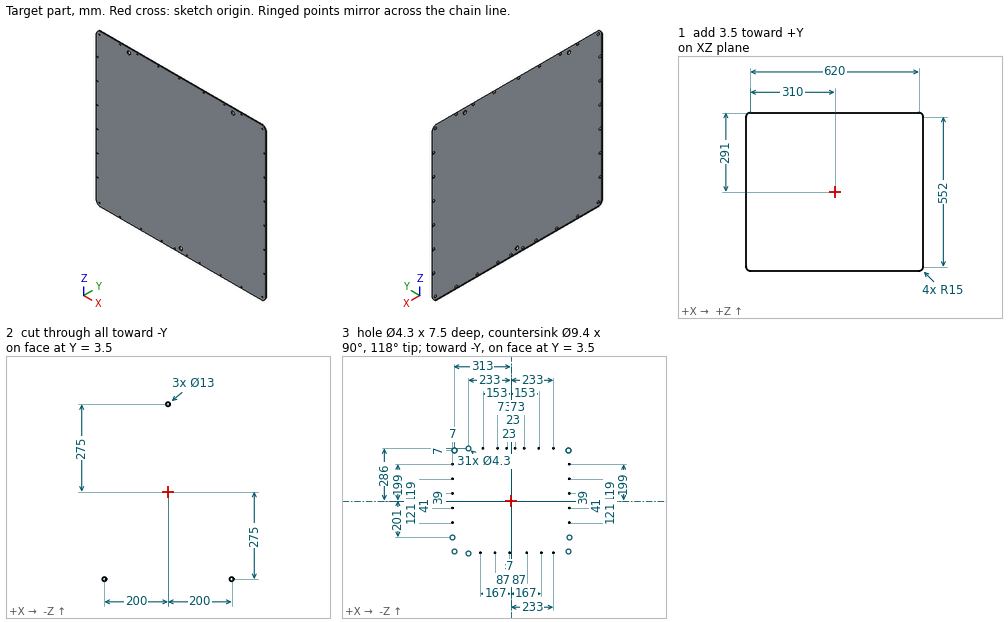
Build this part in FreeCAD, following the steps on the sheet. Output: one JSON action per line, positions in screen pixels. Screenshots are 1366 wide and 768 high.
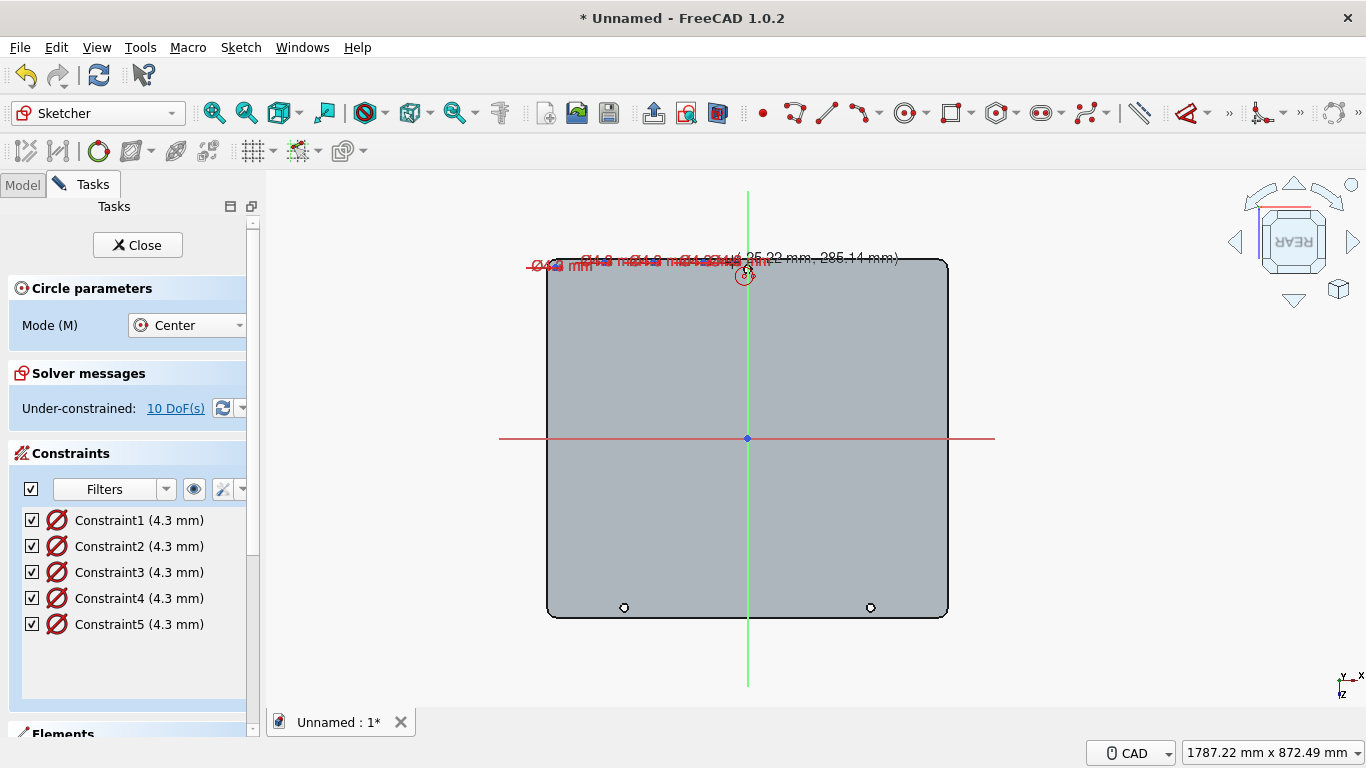
{"action": "scroll", "coordinate": [792, 262], "scroll_direction": "up", "scroll_amount": 15}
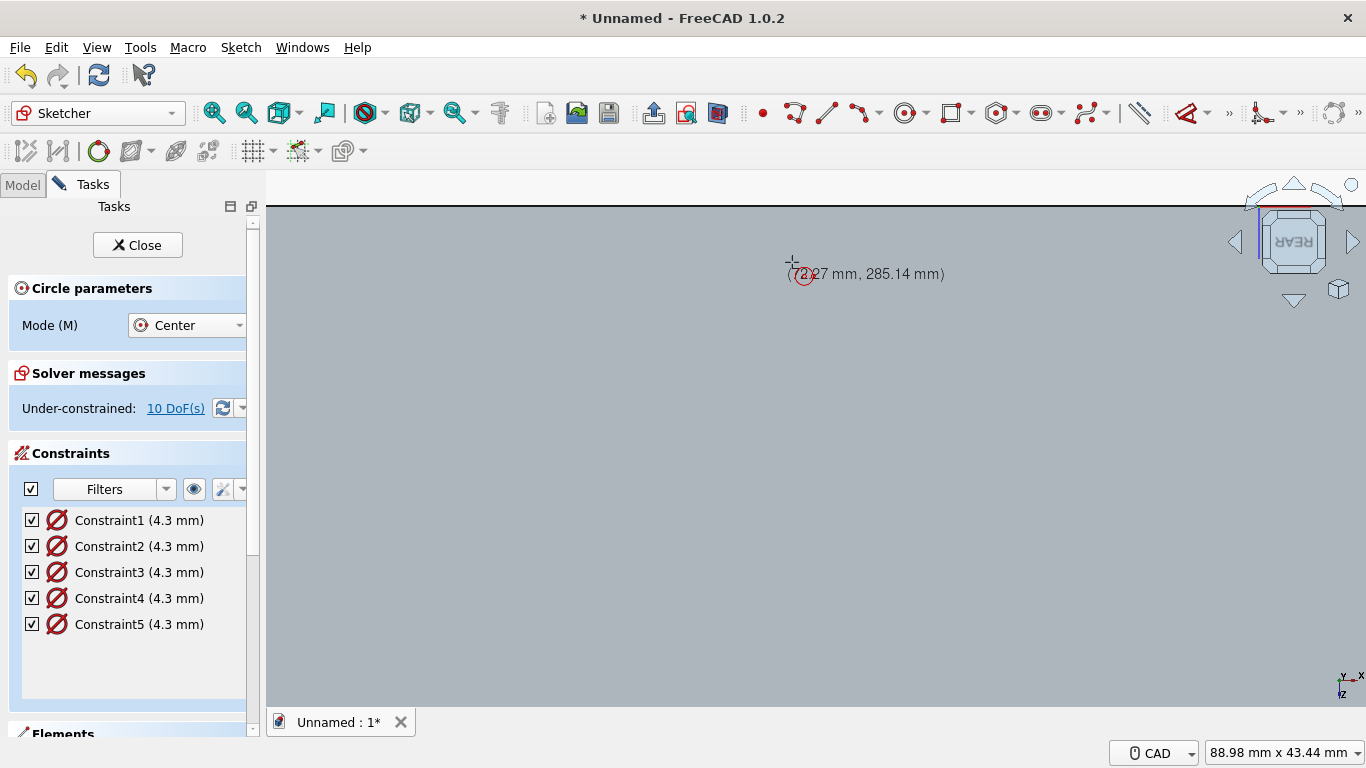
{"action": "scroll", "coordinate": [792, 262], "scroll_direction": "down", "scroll_amount": 15}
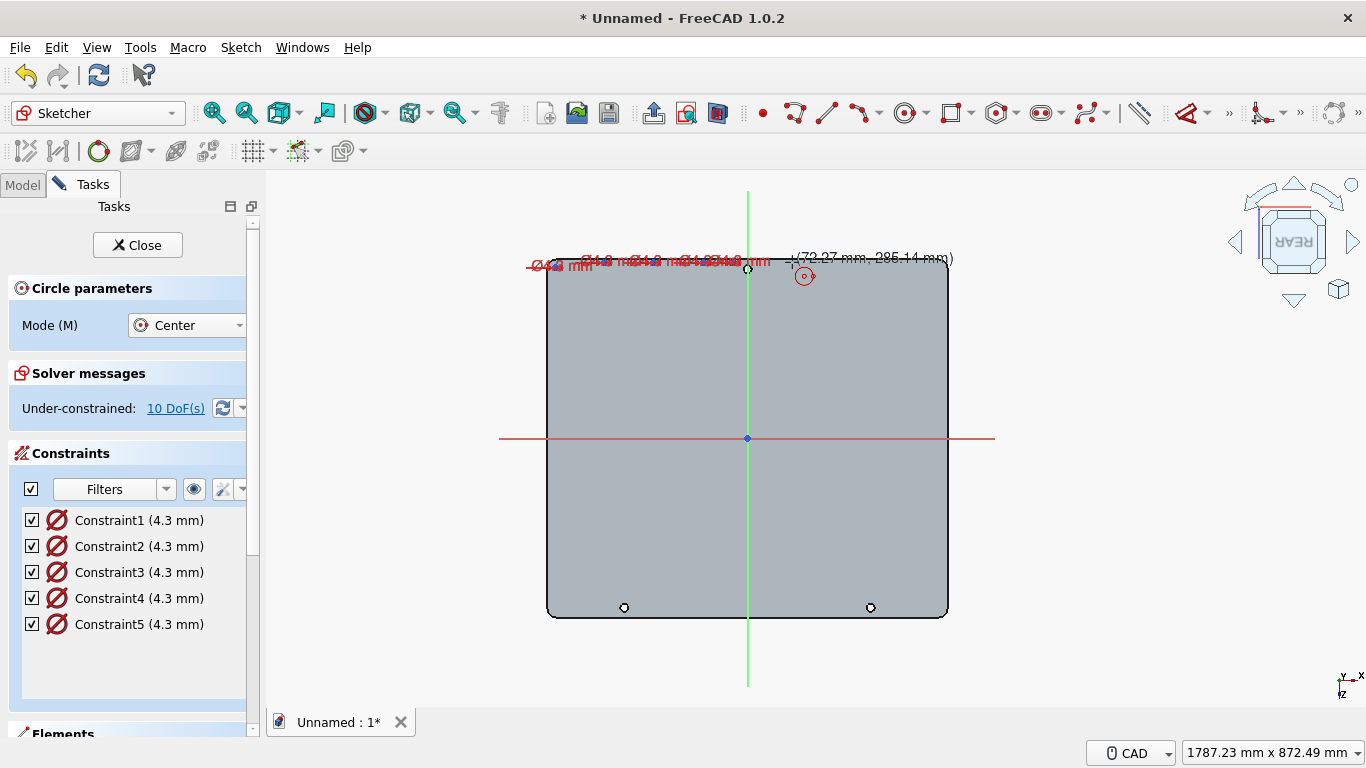
{"action": "left_click", "coordinate": [792, 262]}
{"action": "mouse_move", "coordinate": [793, 262]}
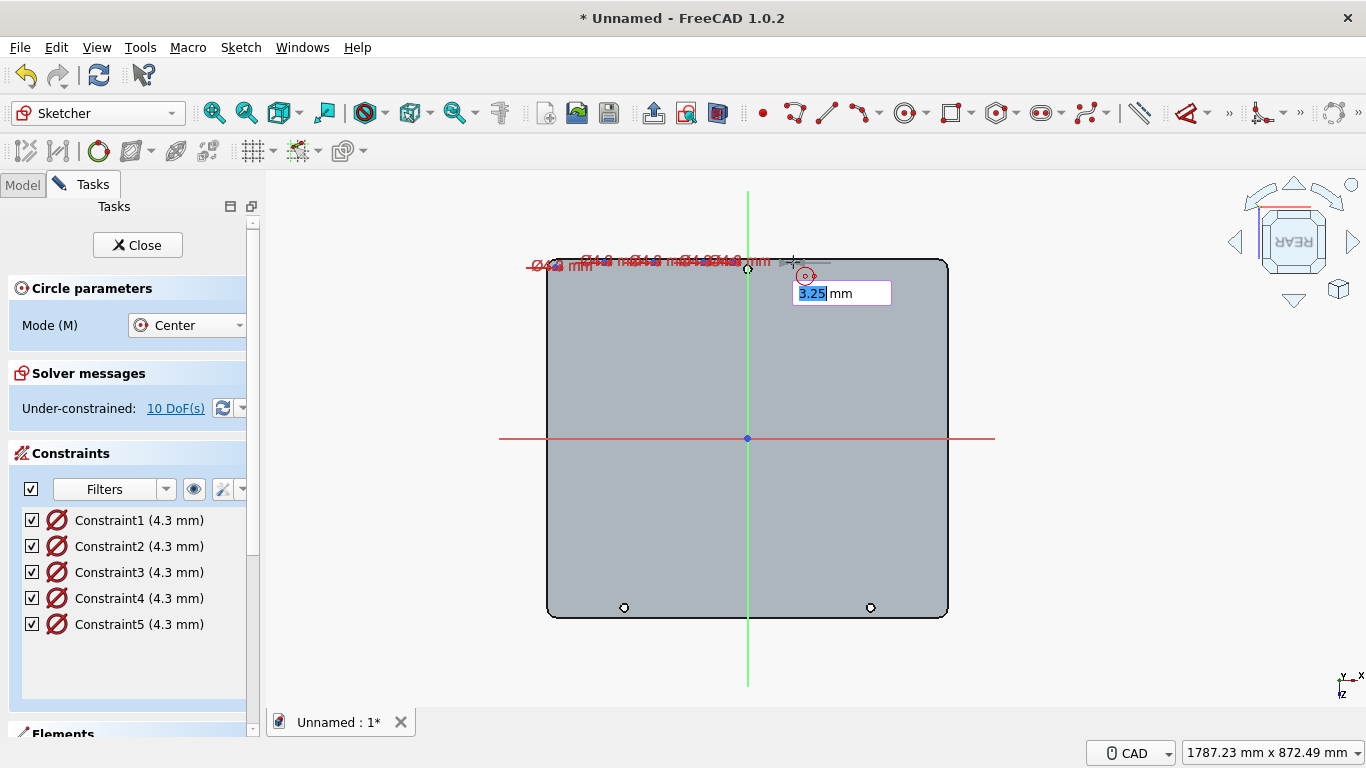
{"action": "type", "text": "4.3"}
{"action": "key", "text": "Return"}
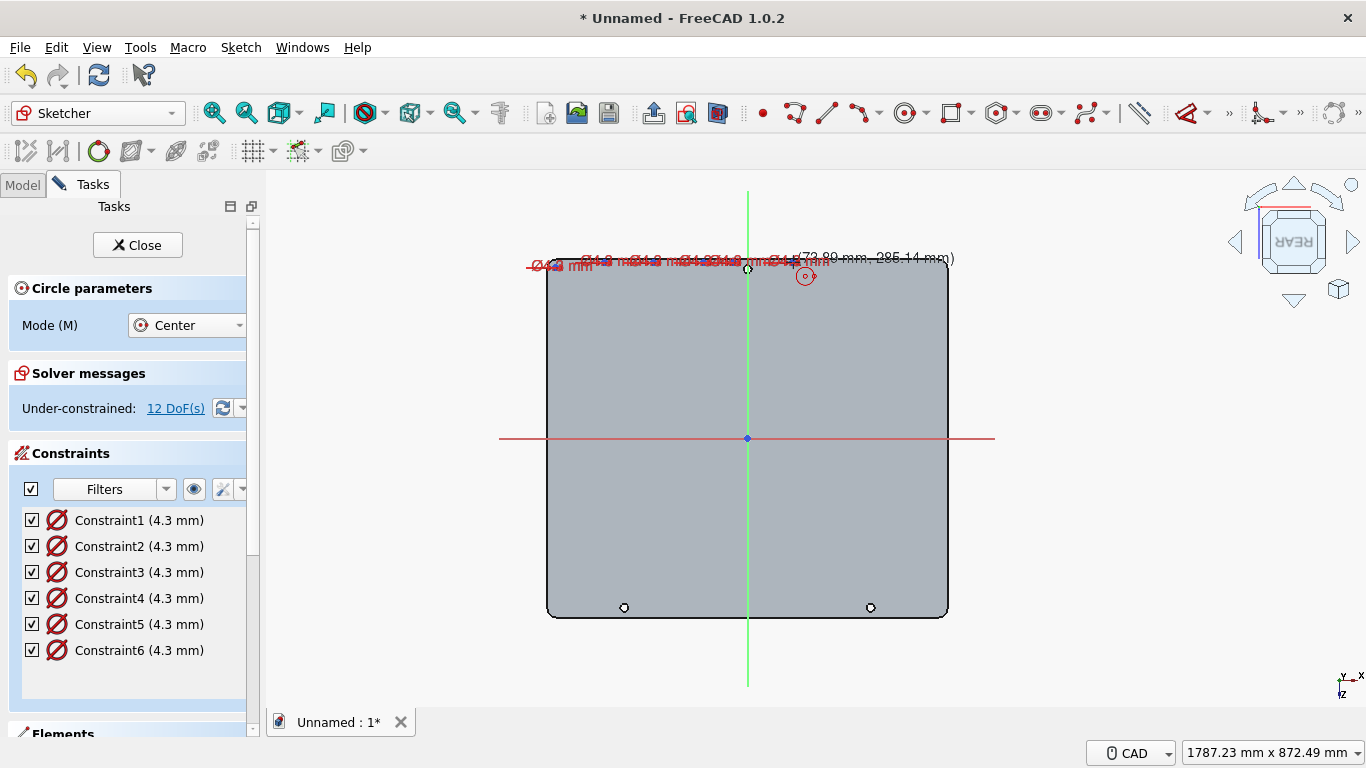
{"action": "scroll", "coordinate": [842, 262], "scroll_direction": "up", "scroll_amount": 15}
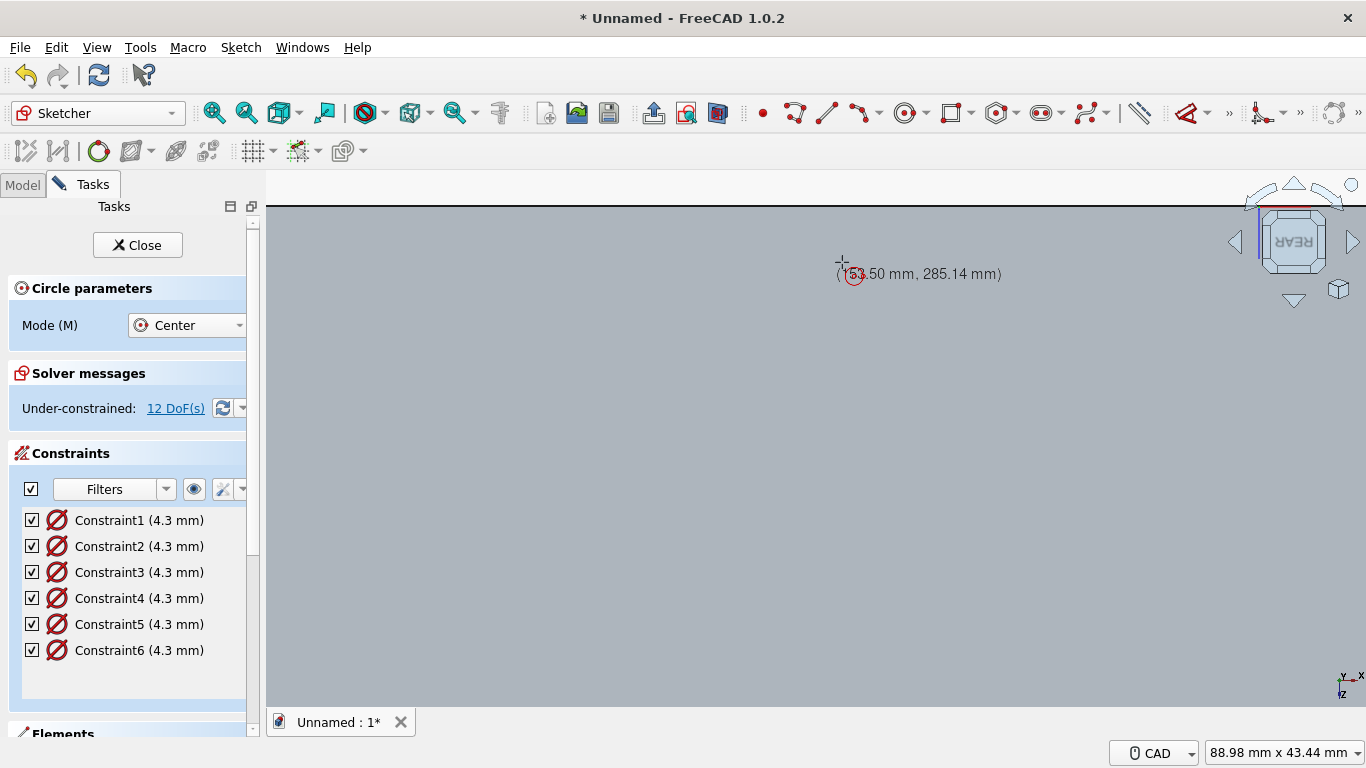
{"action": "scroll", "coordinate": [843, 262], "scroll_direction": "down", "scroll_amount": 15}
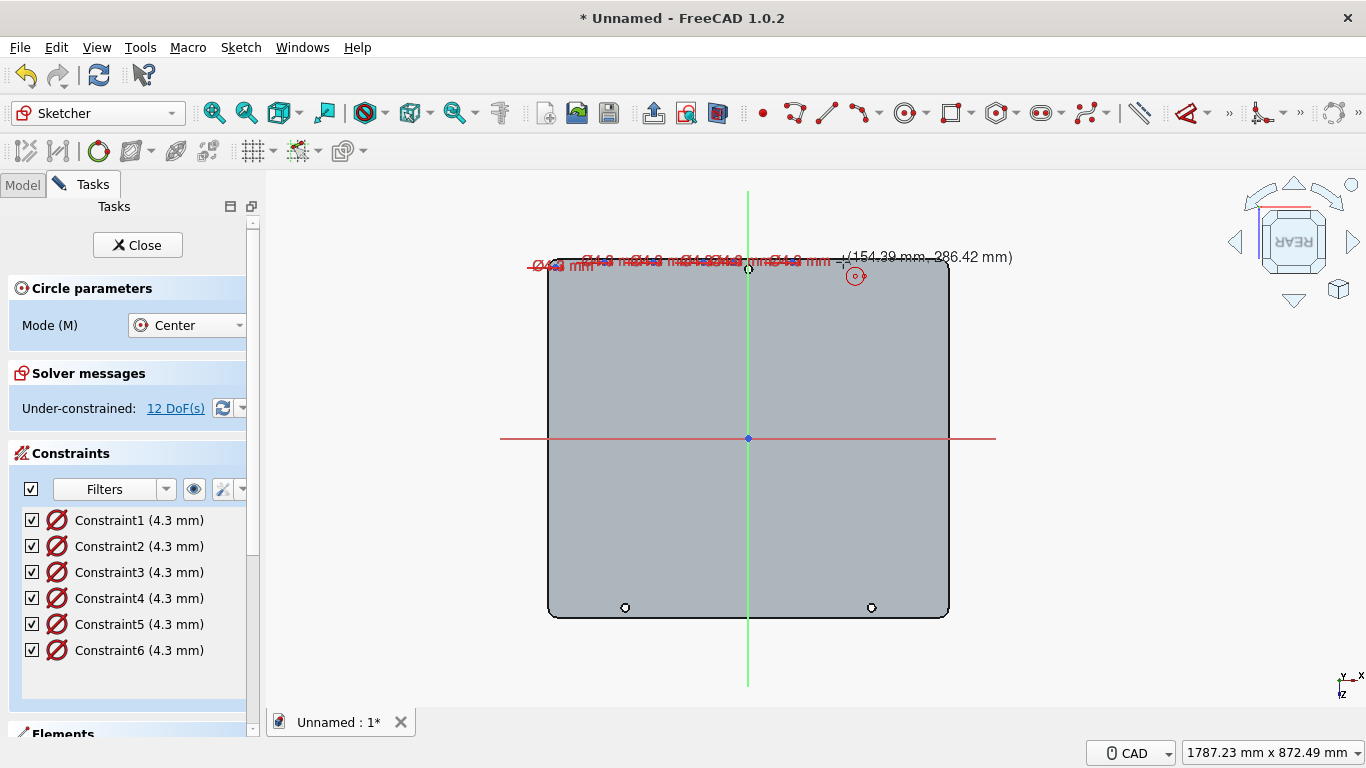
{"action": "left_click", "coordinate": [843, 262]}
{"action": "mouse_move", "coordinate": [844, 262]}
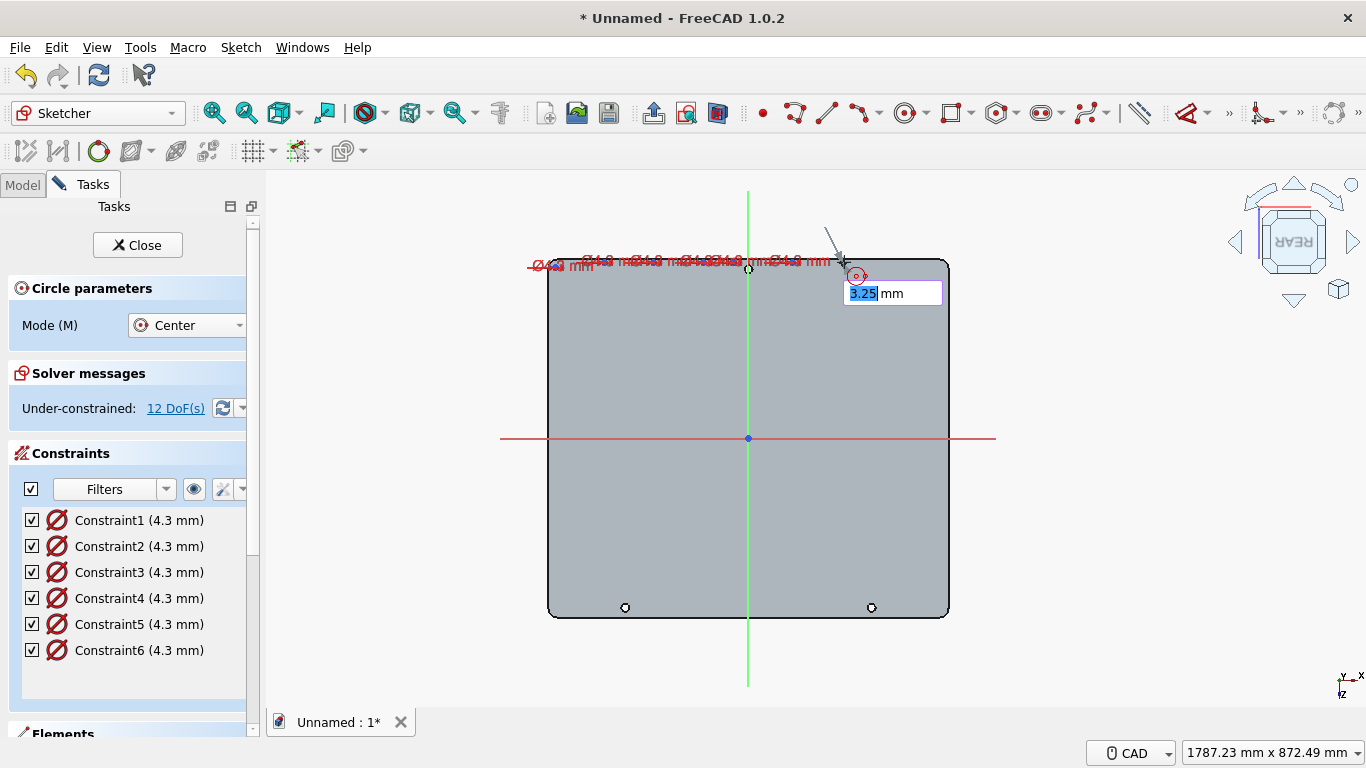
{"action": "type", "text": "4.3"}
{"action": "key", "text": "Return"}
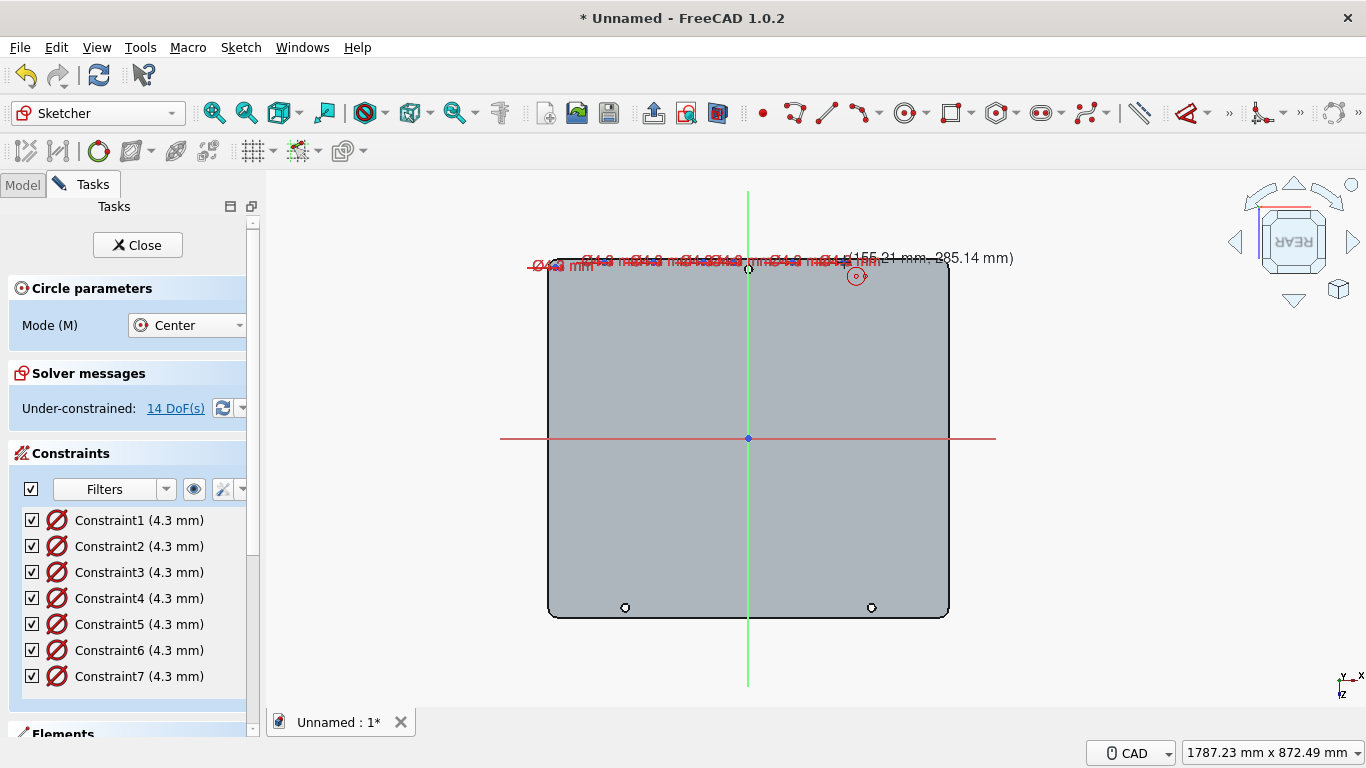
{"action": "scroll", "coordinate": [941, 267], "scroll_direction": "up", "scroll_amount": 15}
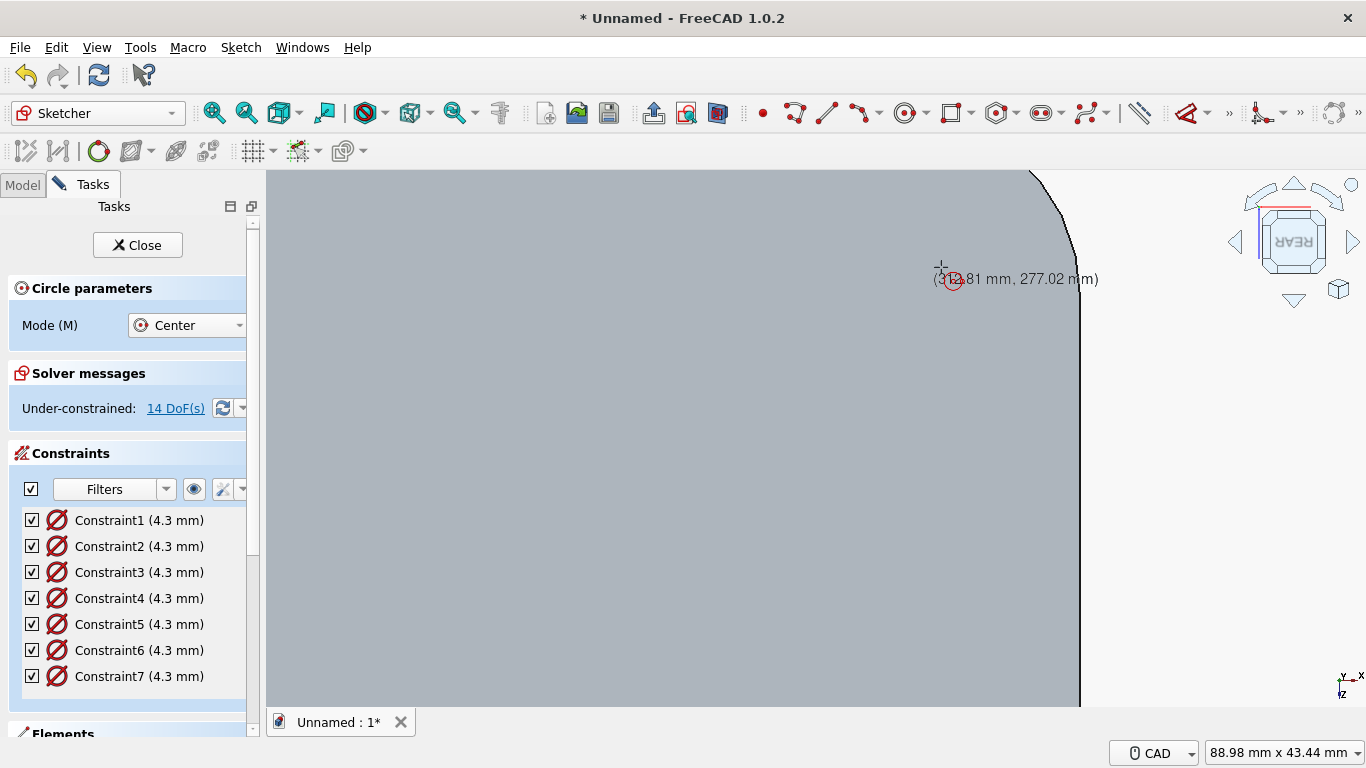
{"action": "scroll", "coordinate": [941, 267], "scroll_direction": "down", "scroll_amount": 15}